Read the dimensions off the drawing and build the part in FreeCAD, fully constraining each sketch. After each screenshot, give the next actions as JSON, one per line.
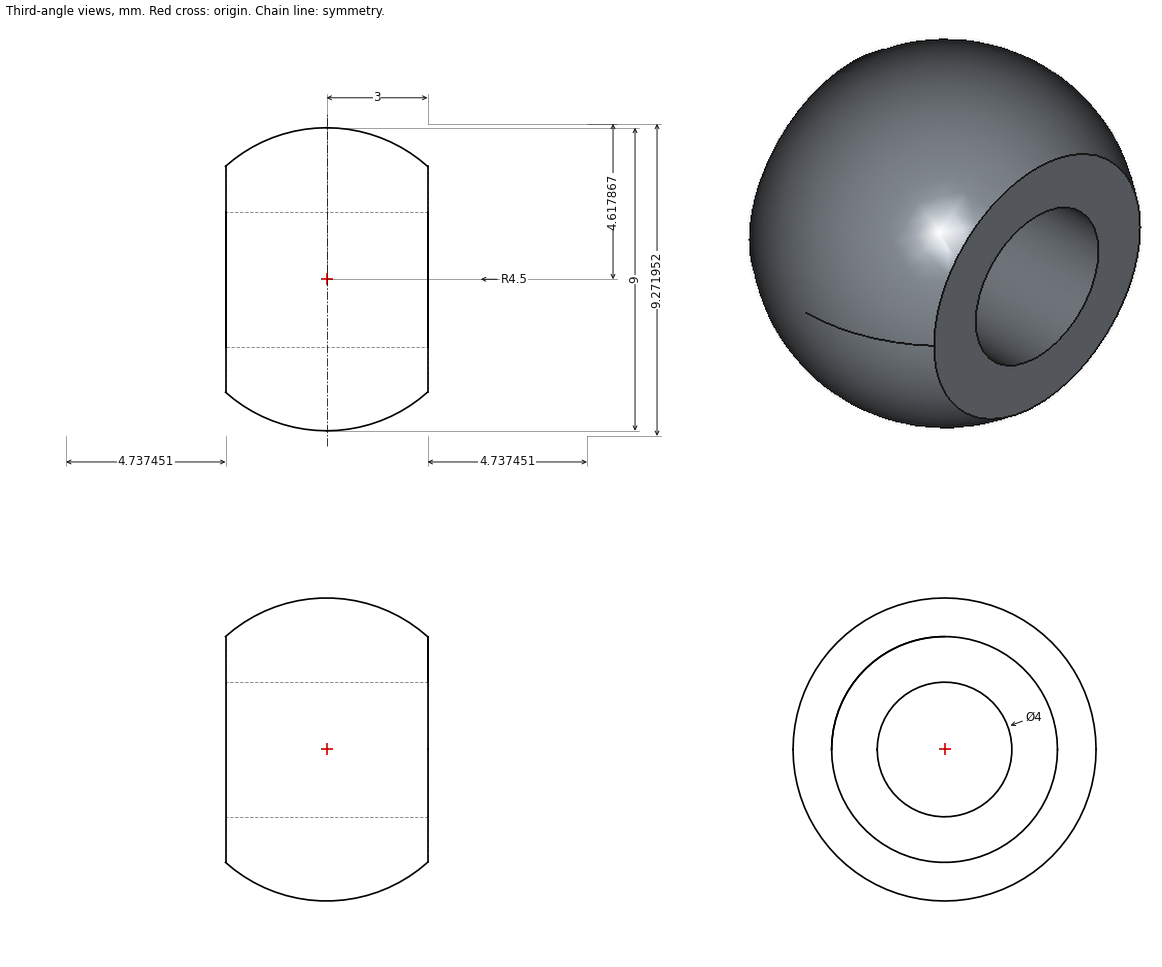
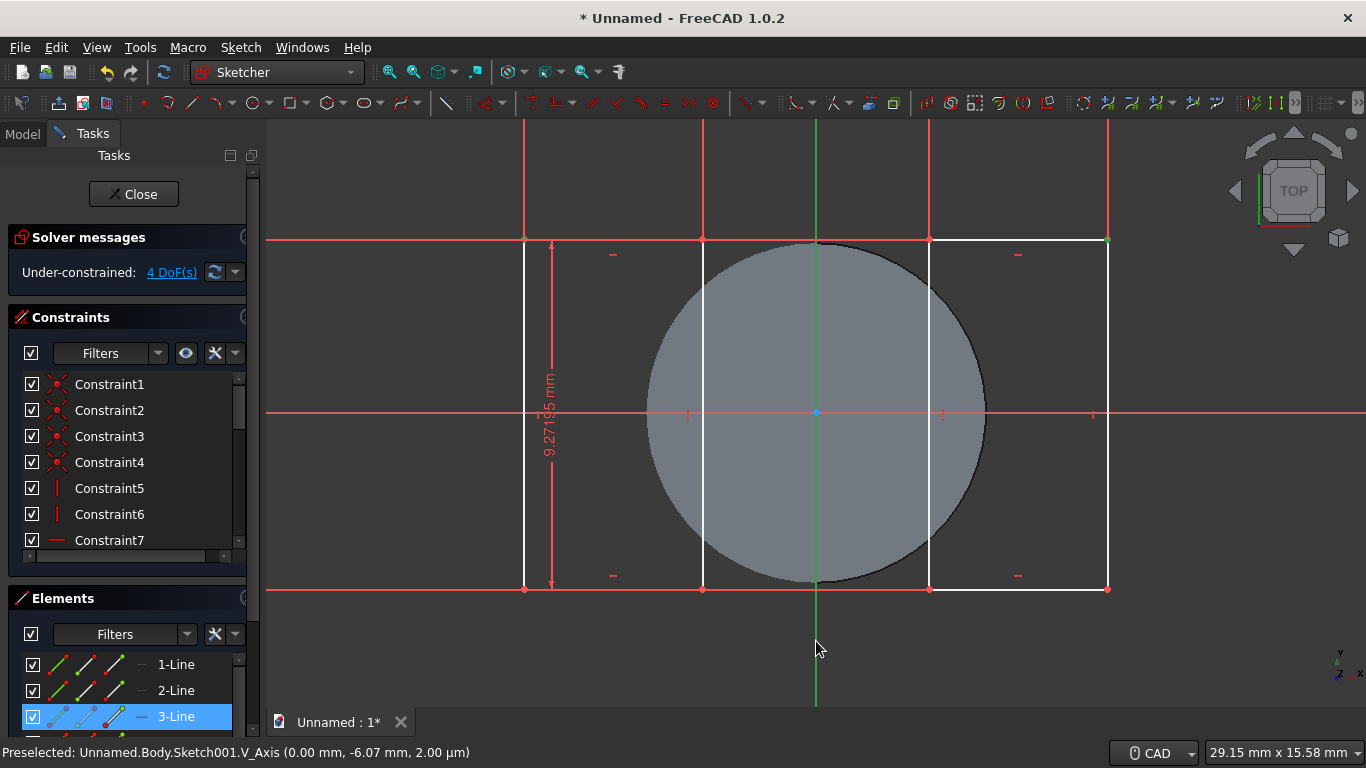
{"action": "key", "text": "s"}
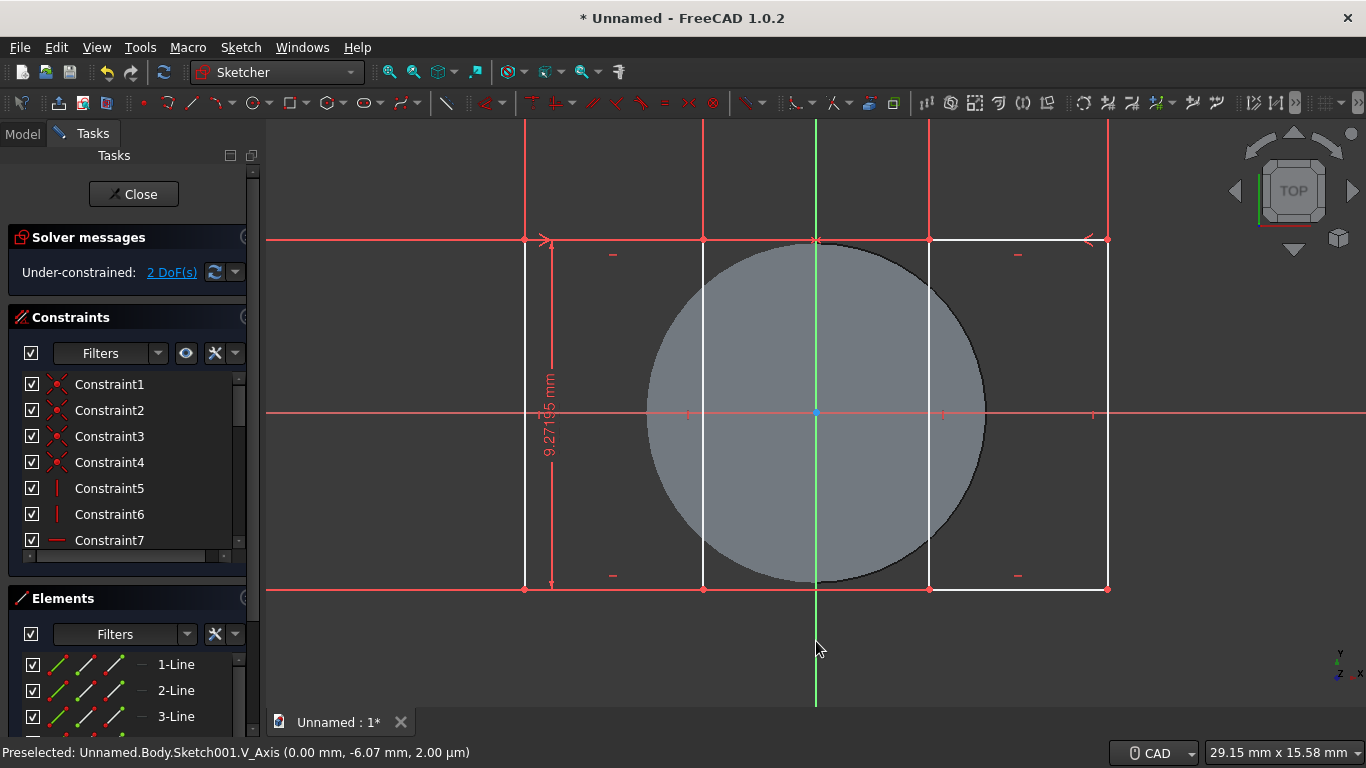
{"action": "left_click", "coordinate": [486, 104]}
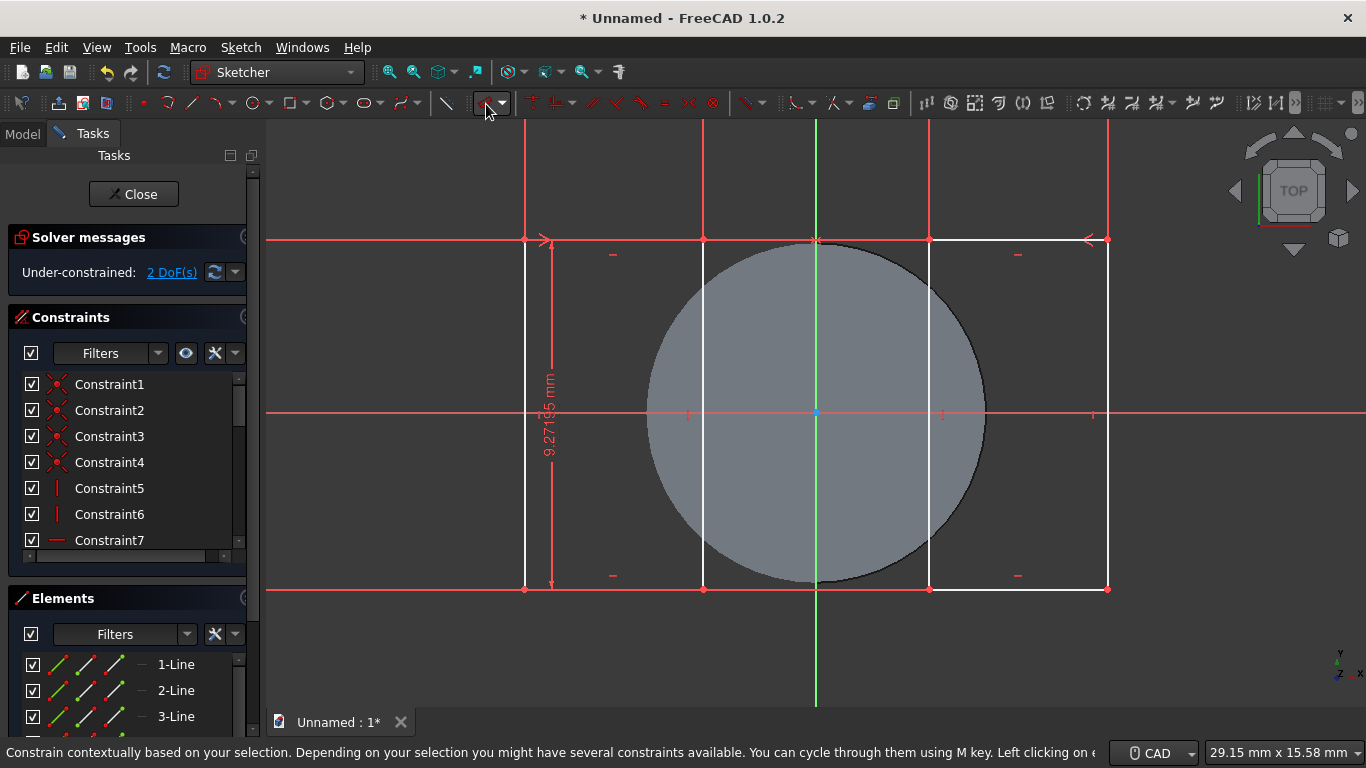
{"action": "left_click", "coordinate": [929, 240]}
{"action": "left_click", "coordinate": [873, 206]}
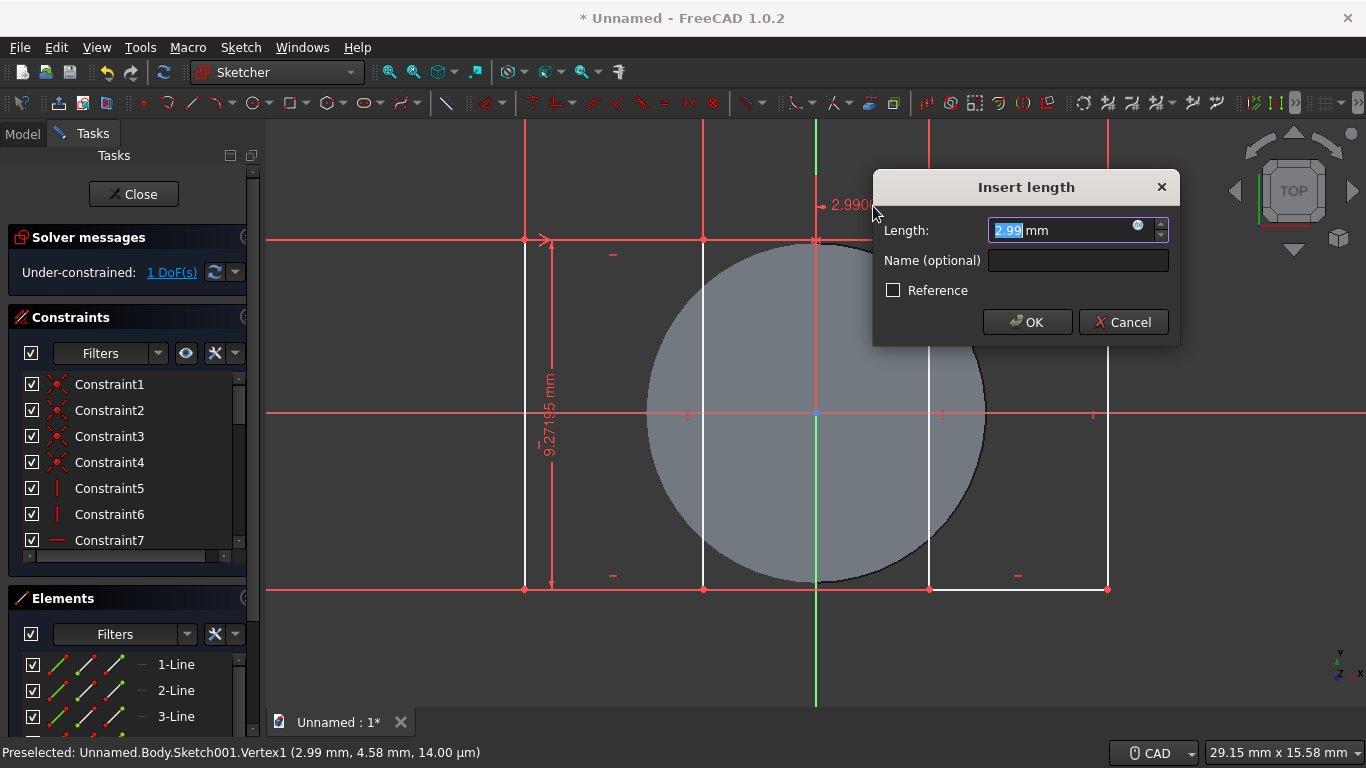
{"action": "type", "text": "3"}
{"action": "key", "text": "Return"}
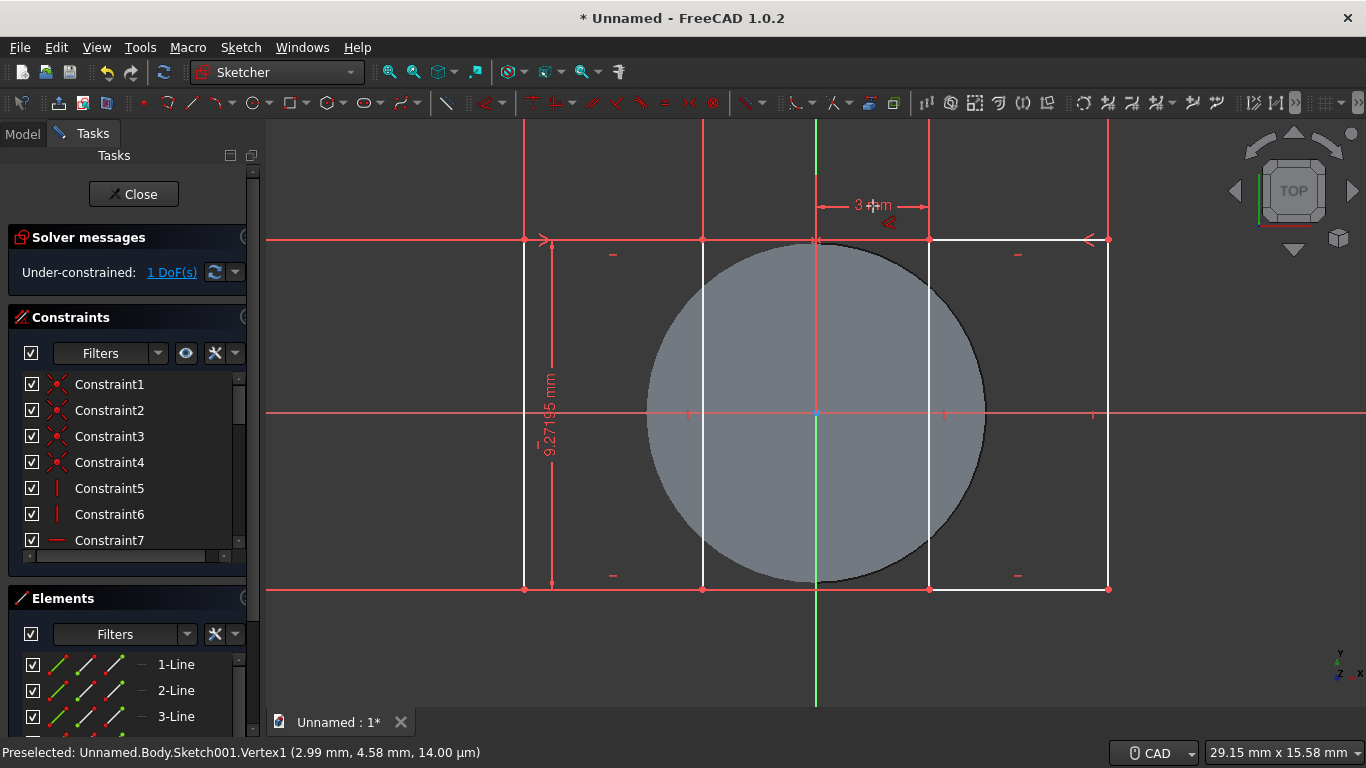
{"action": "left_click", "coordinate": [929, 240]}
{"action": "left_click", "coordinate": [963, 326]}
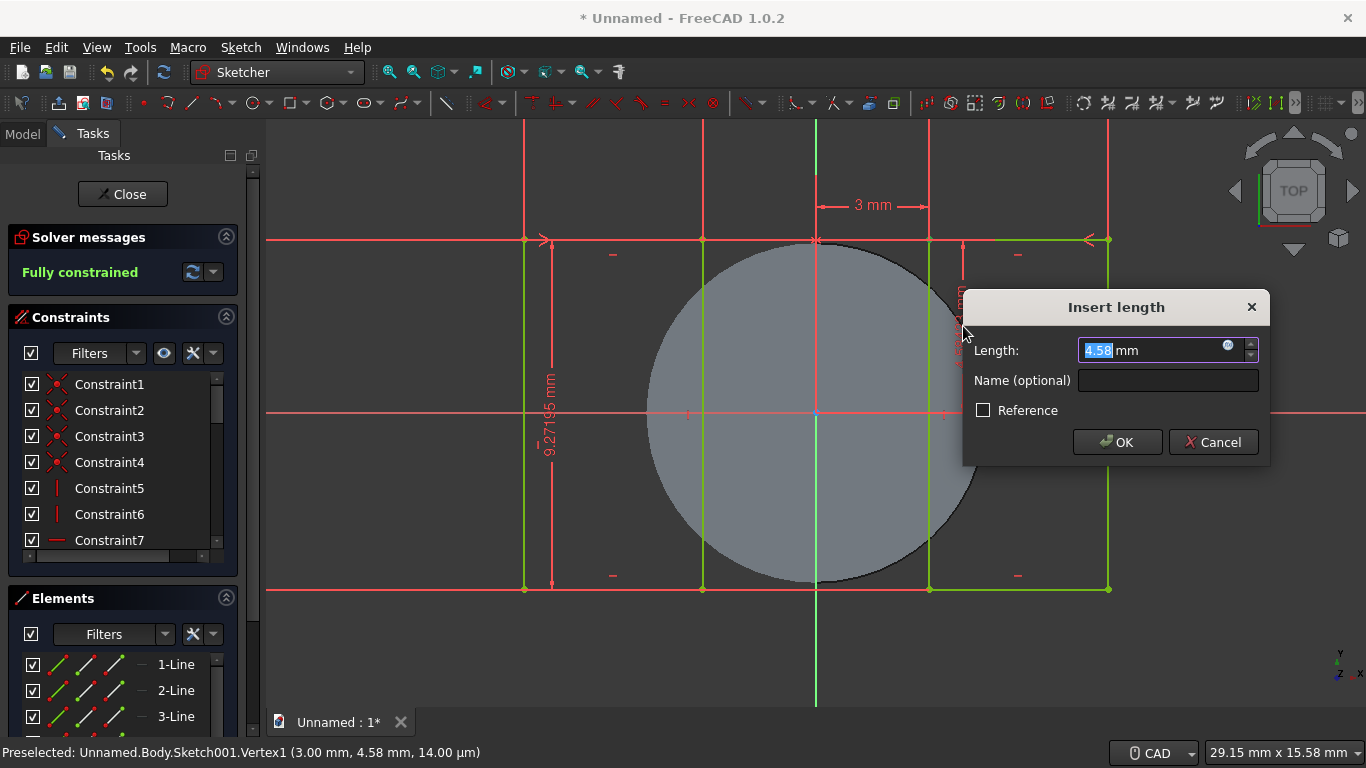
{"action": "type", "text": "4.617867"}
{"action": "key", "text": "Return"}
{"action": "key", "text": "Escape"}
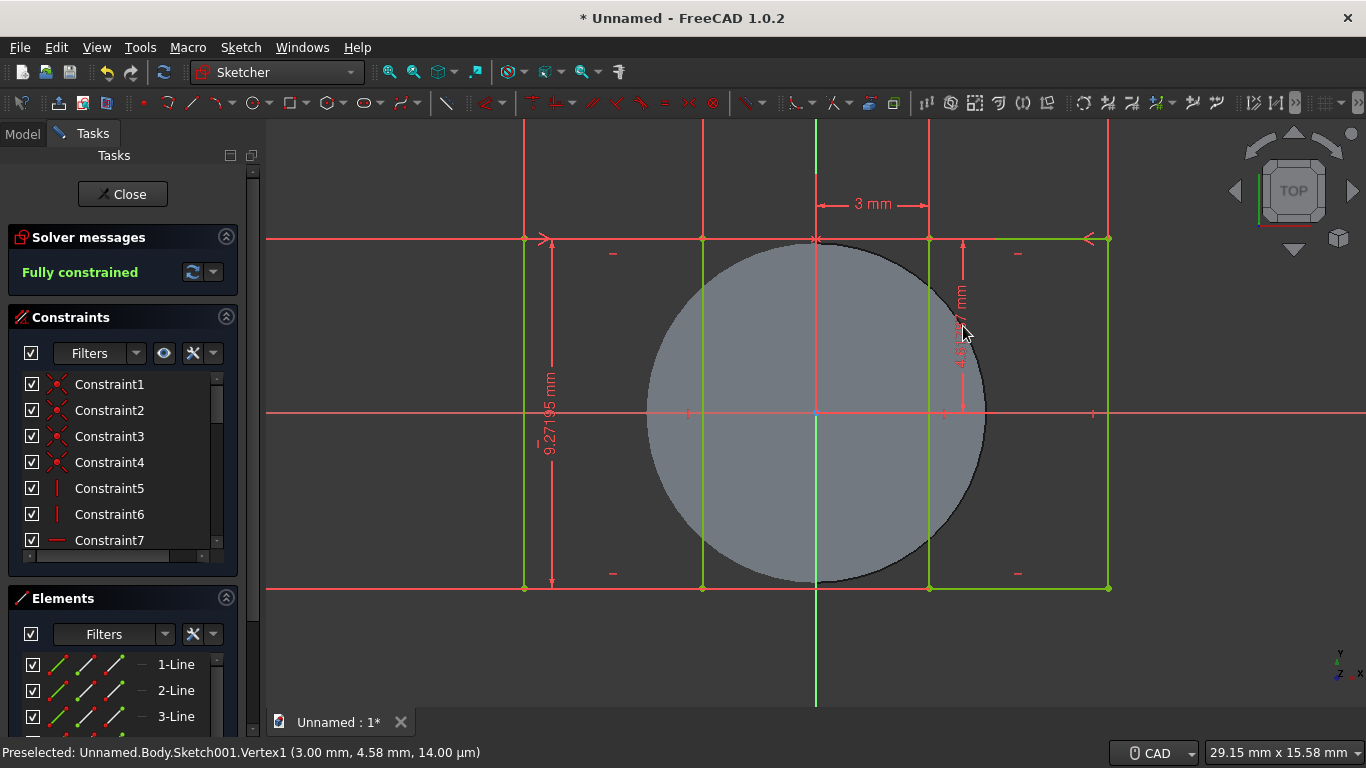
{"action": "left_click", "coordinate": [123, 194]}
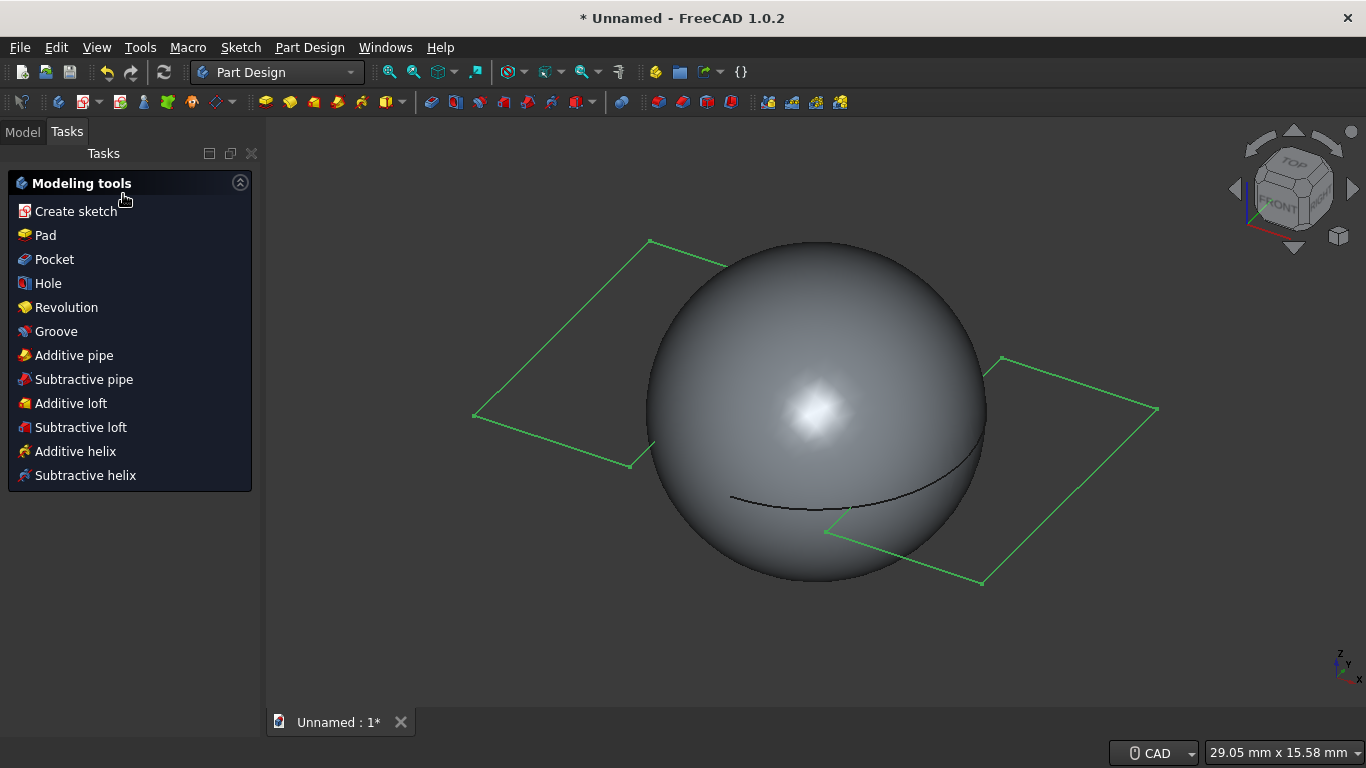
{"action": "left_click", "coordinate": [432, 102]}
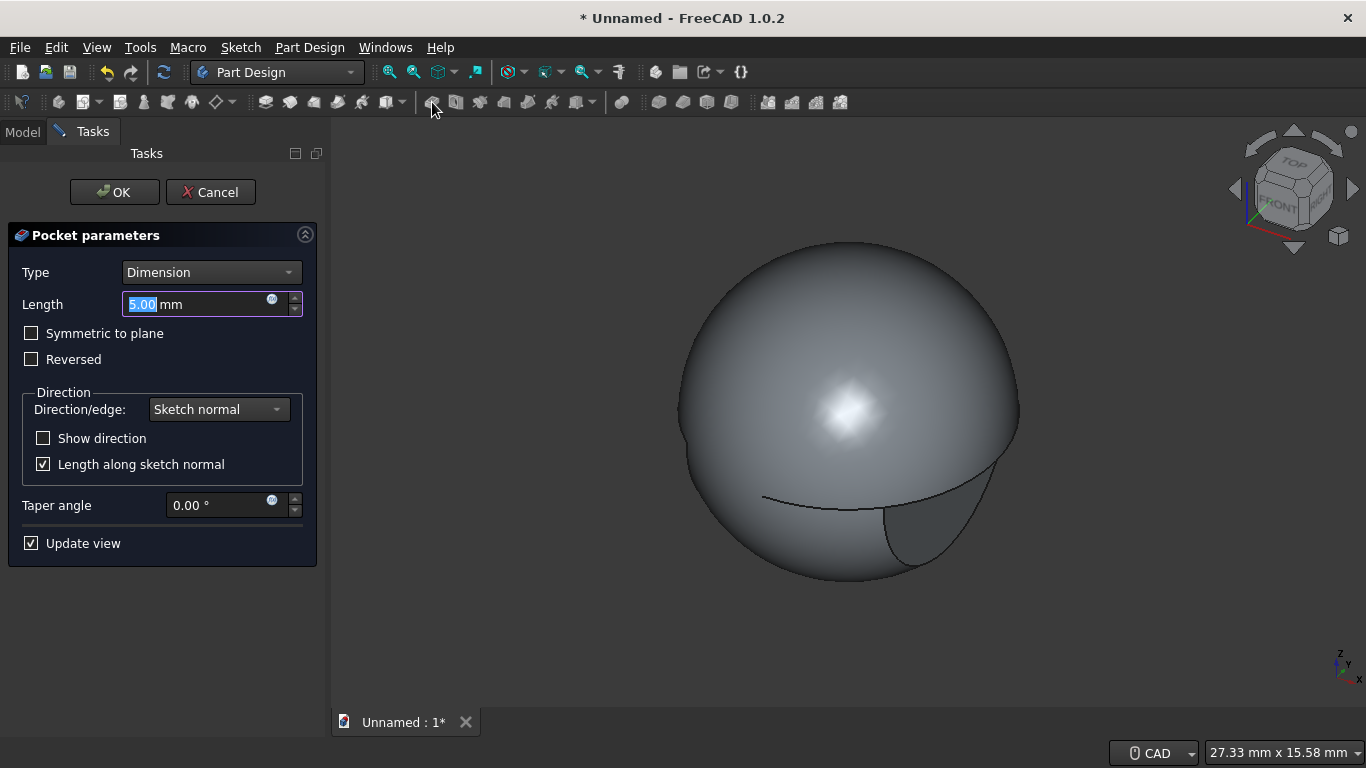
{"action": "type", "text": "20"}
{"action": "key", "text": "Tab"}